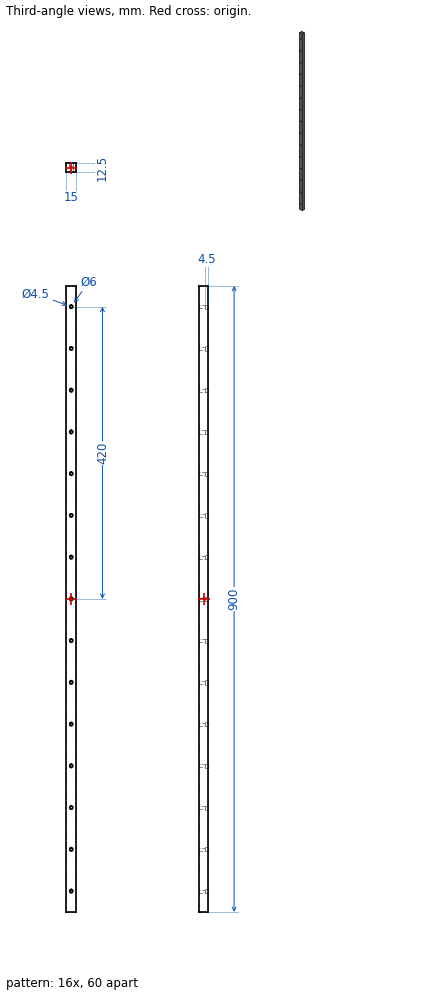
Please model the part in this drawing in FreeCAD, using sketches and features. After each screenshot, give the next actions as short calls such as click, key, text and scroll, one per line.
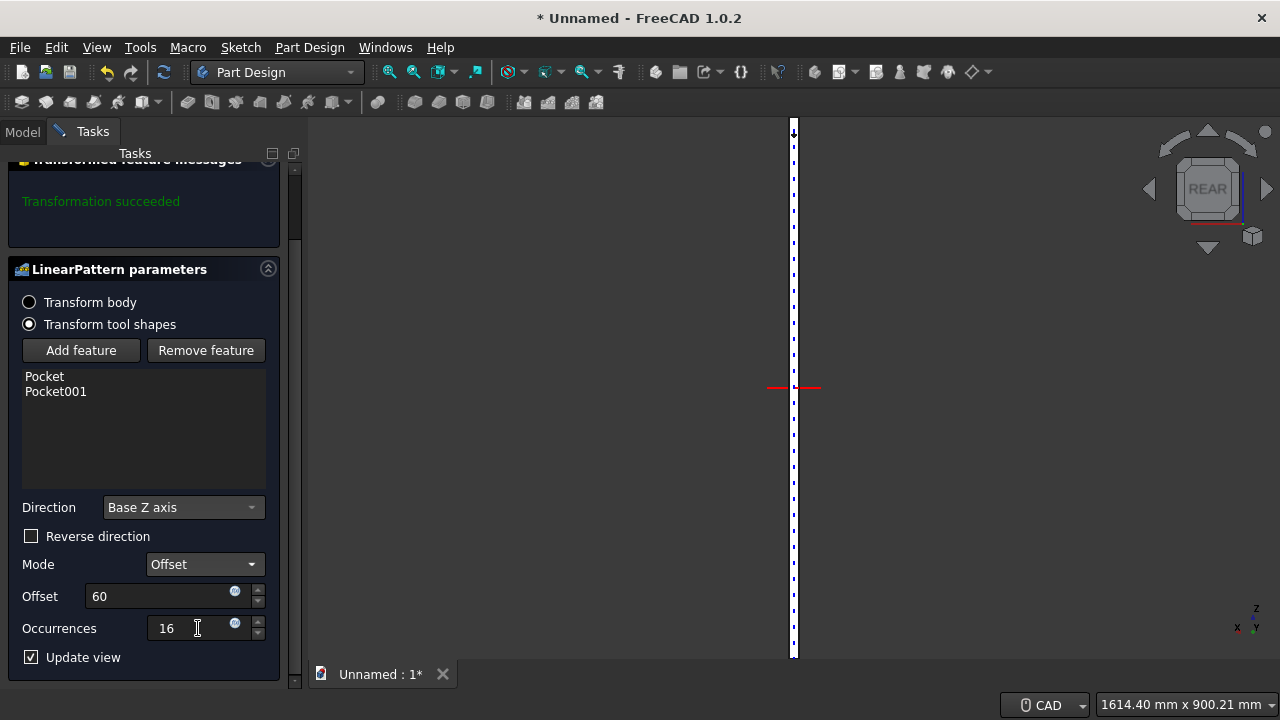
click(30, 536)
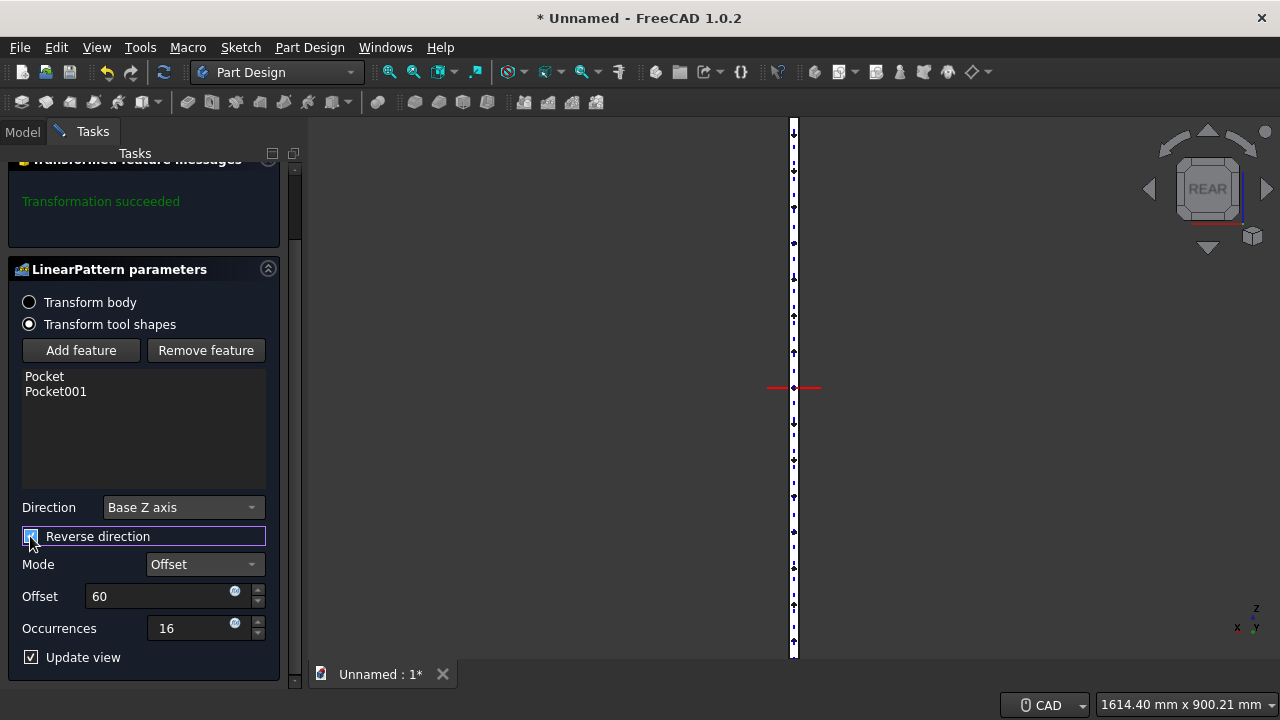
scroll(295, 426, up, 3)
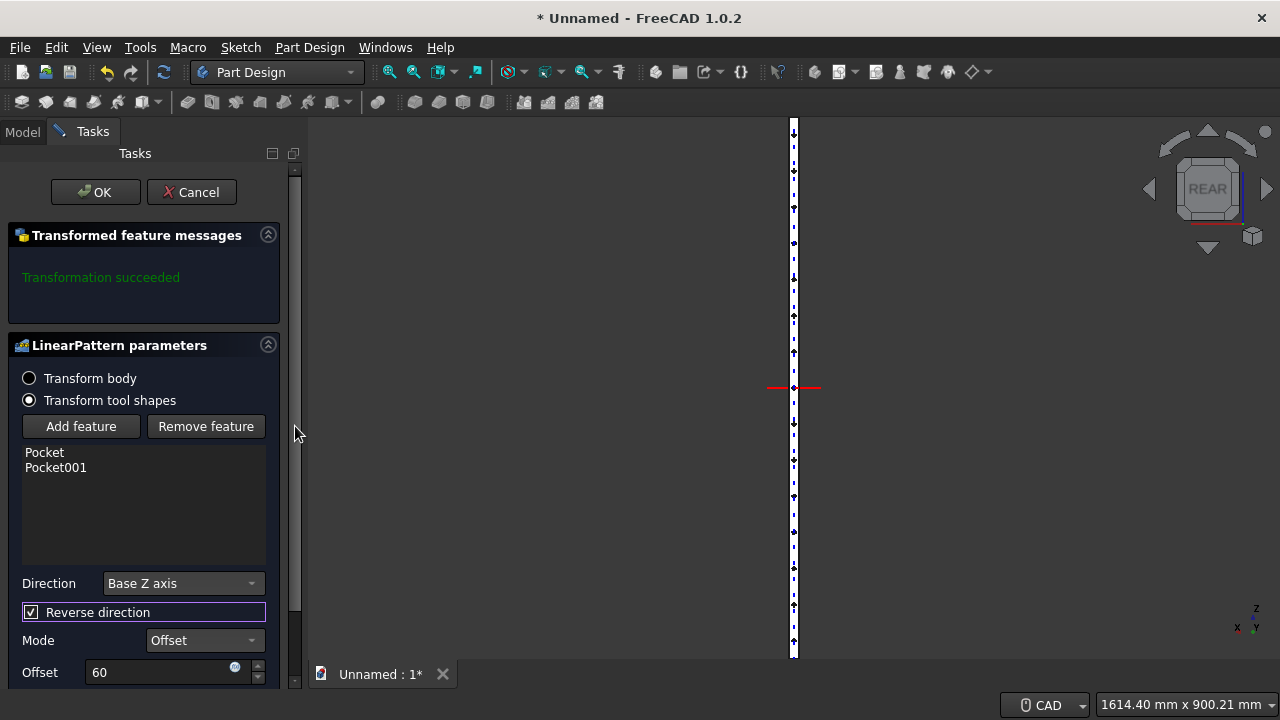
click(96, 192)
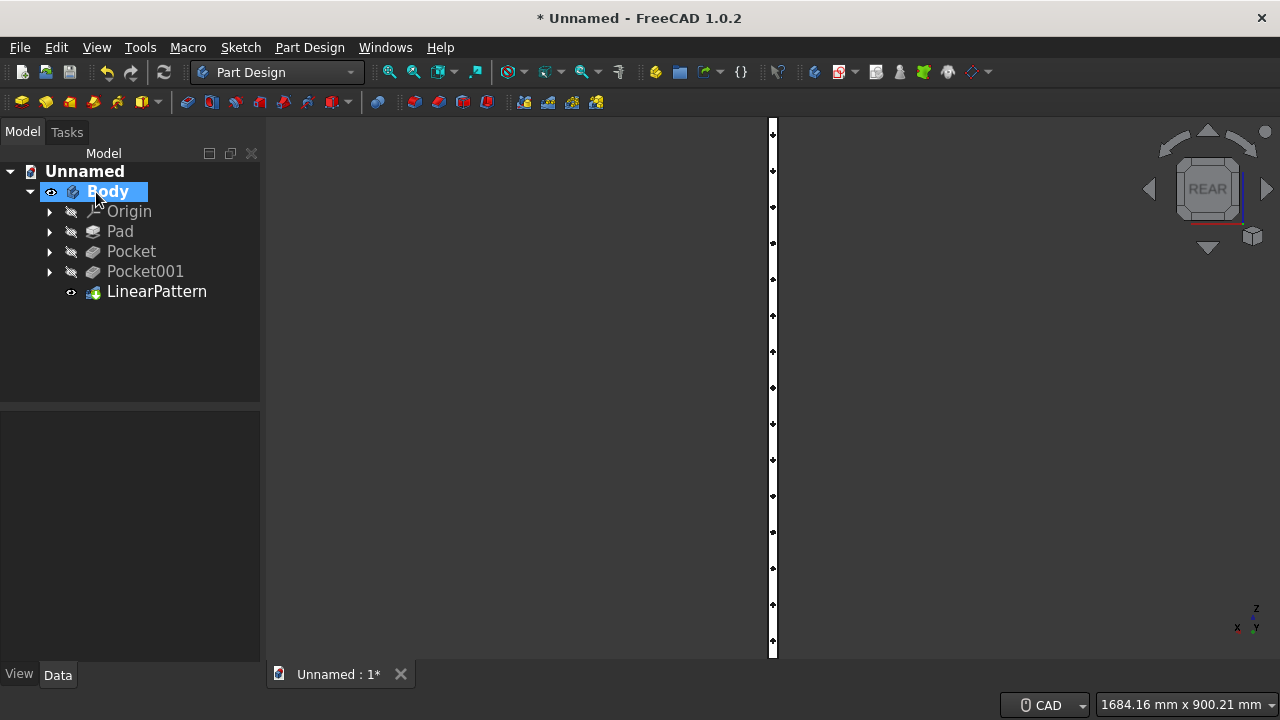
key(0)